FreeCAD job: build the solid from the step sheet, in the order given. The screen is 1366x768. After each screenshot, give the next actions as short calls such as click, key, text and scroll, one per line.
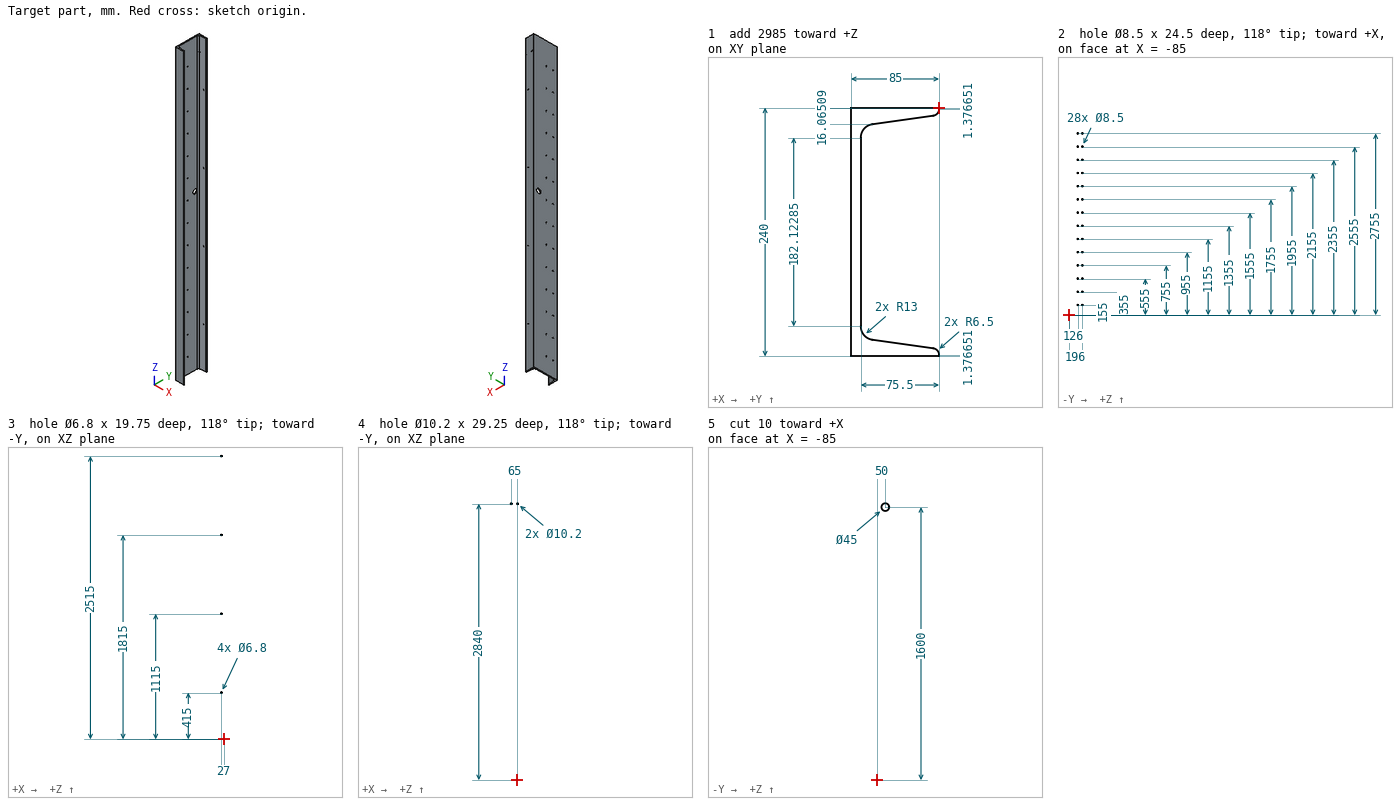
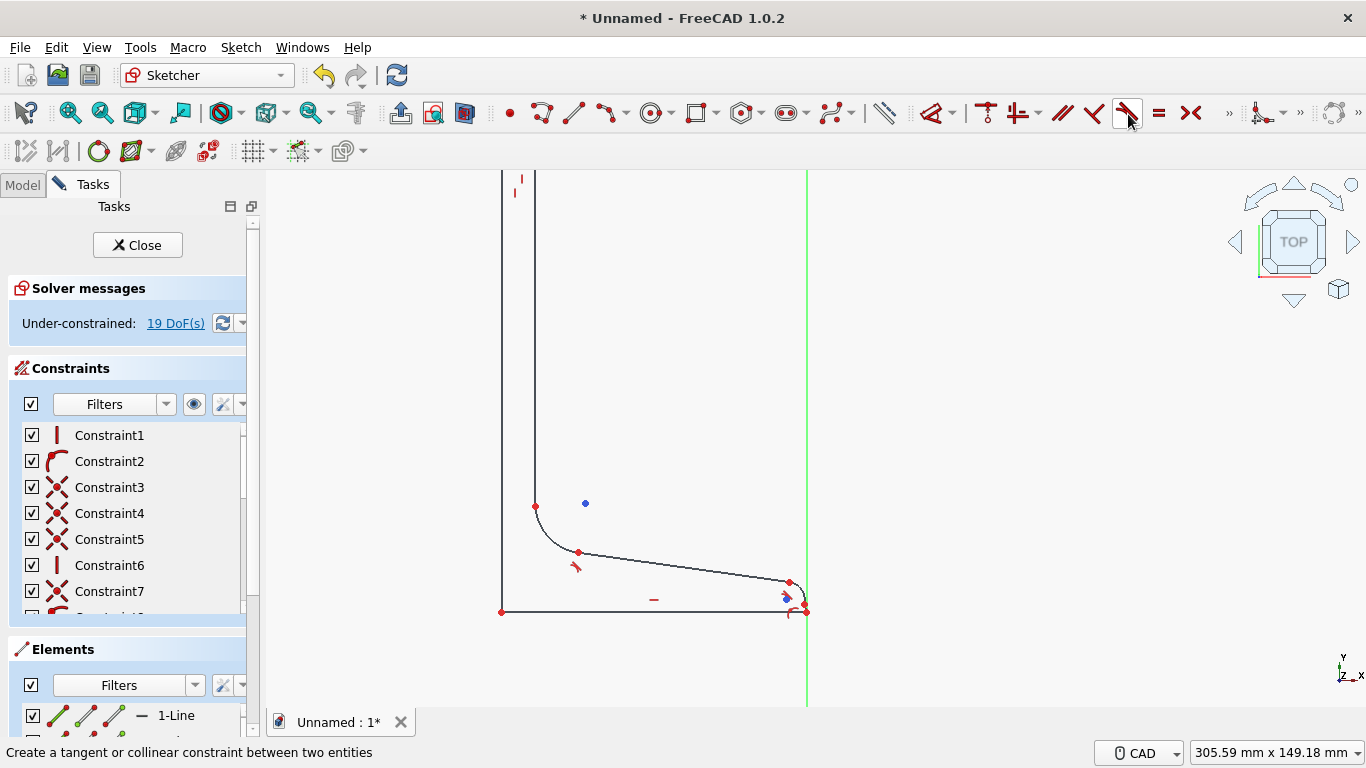
click(535, 310)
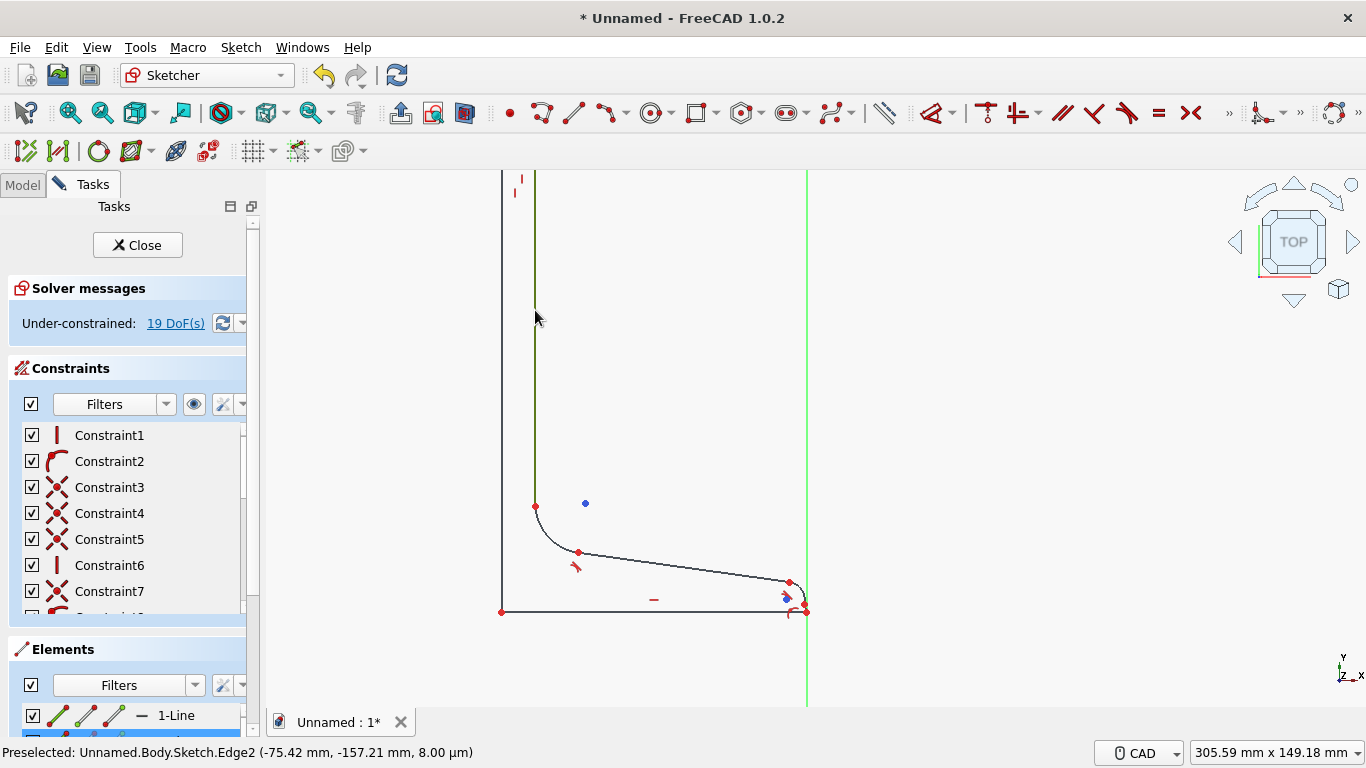
click(541, 526)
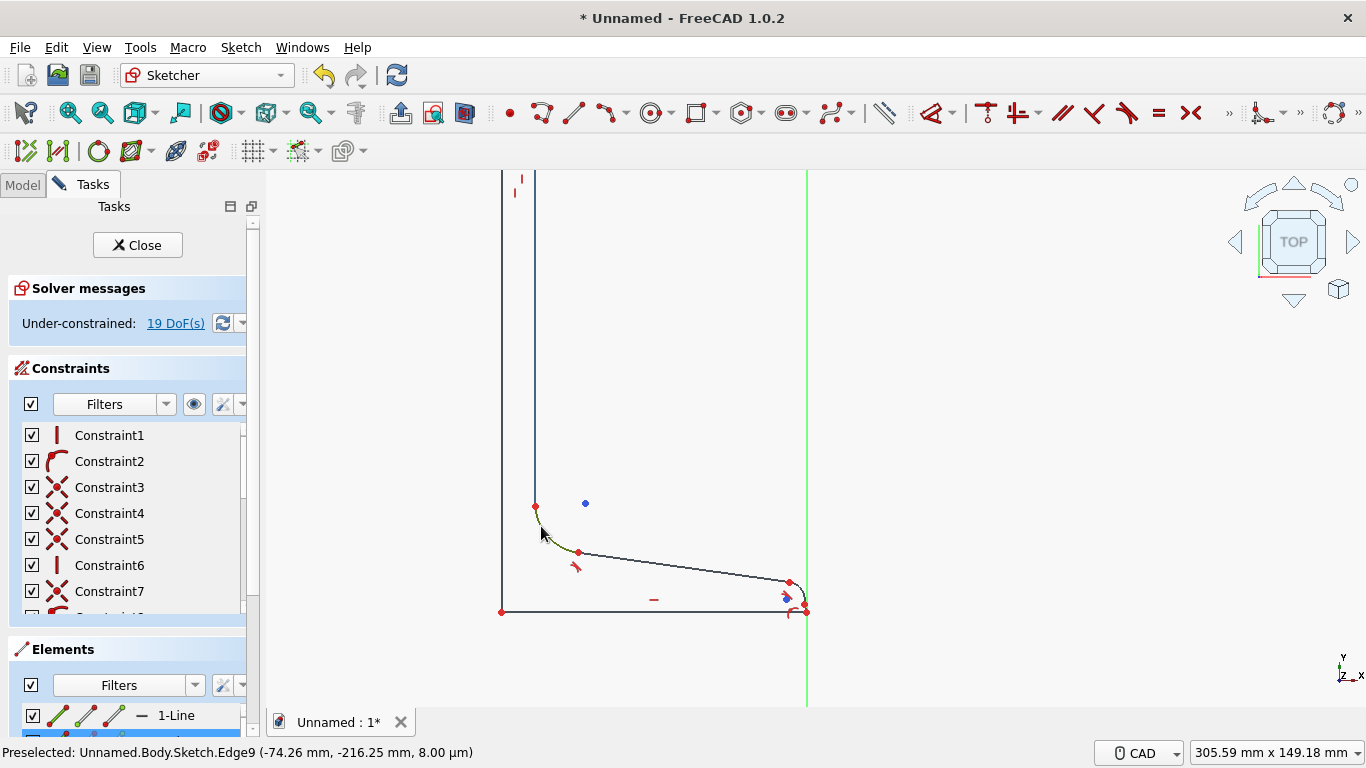
click(1128, 114)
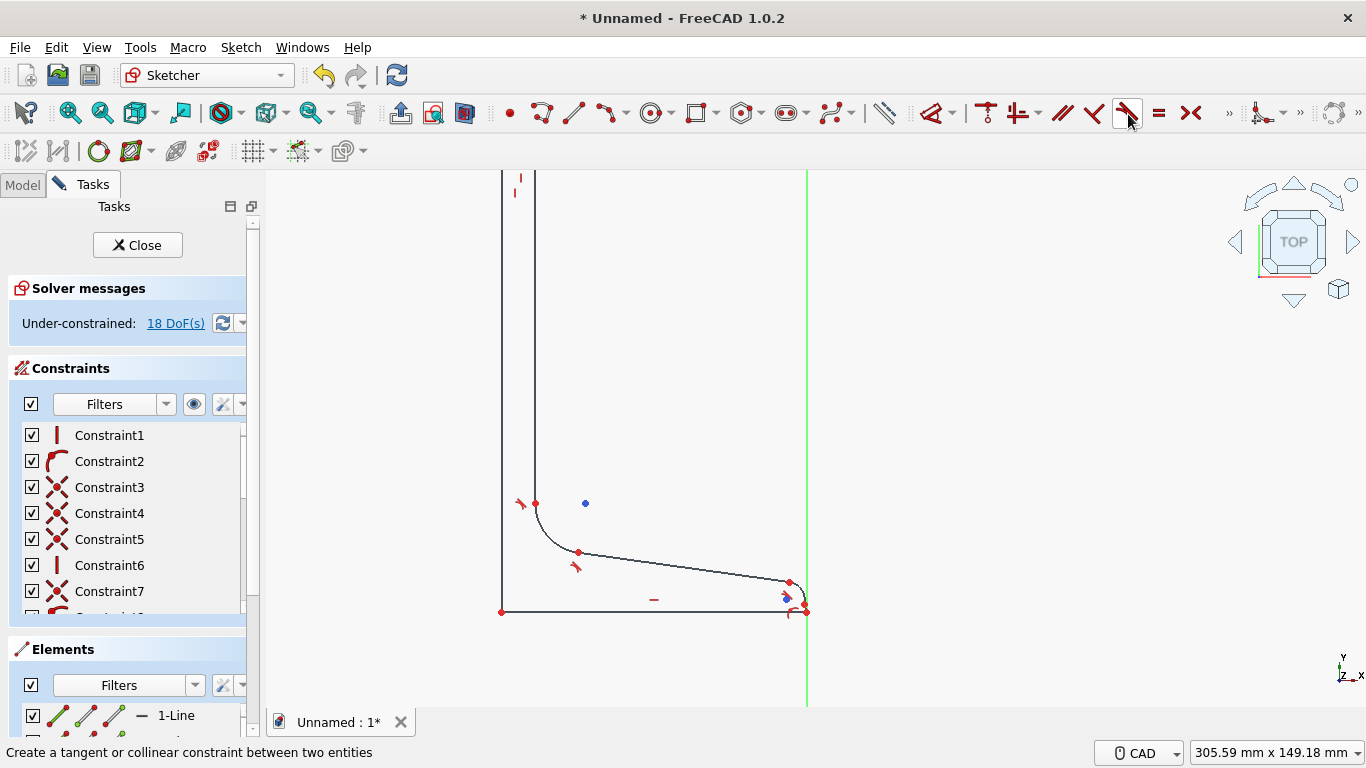
click(535, 308)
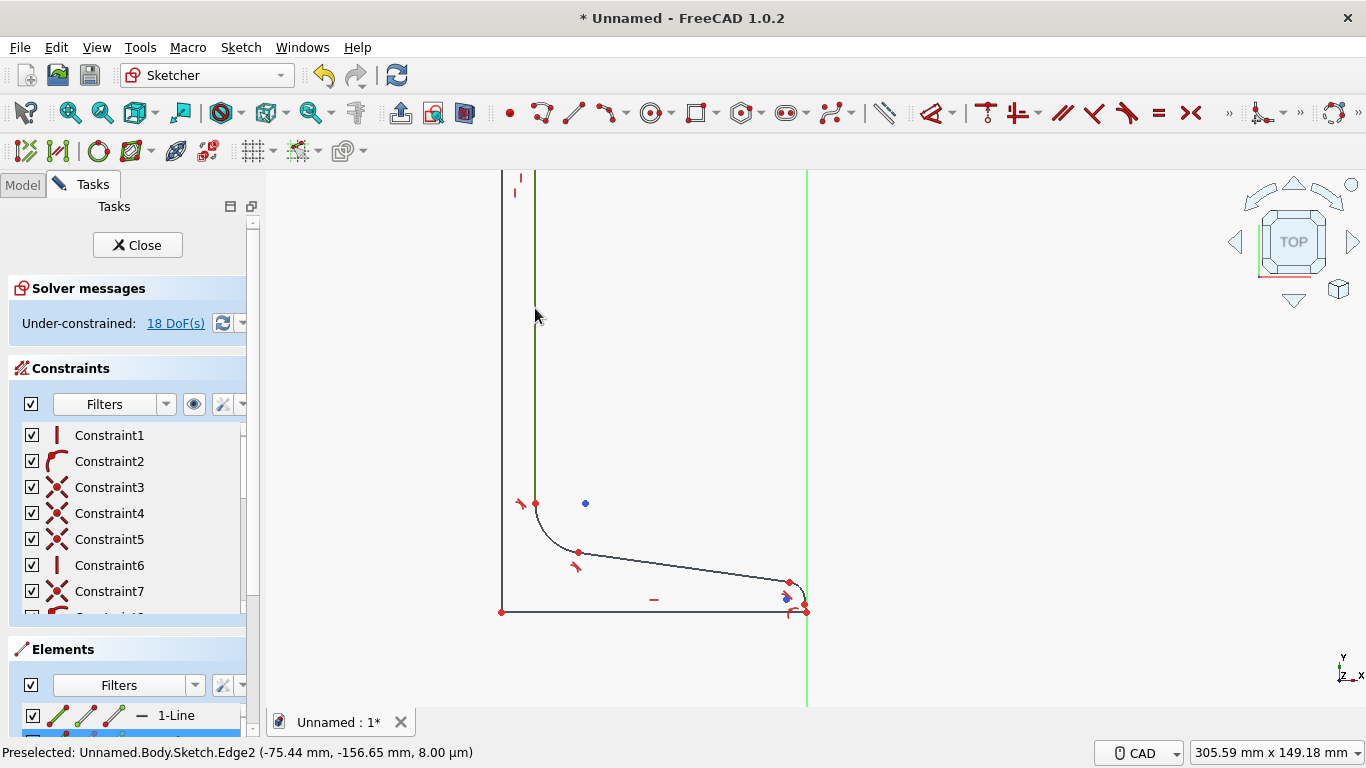
scroll(802, 591, down, 5)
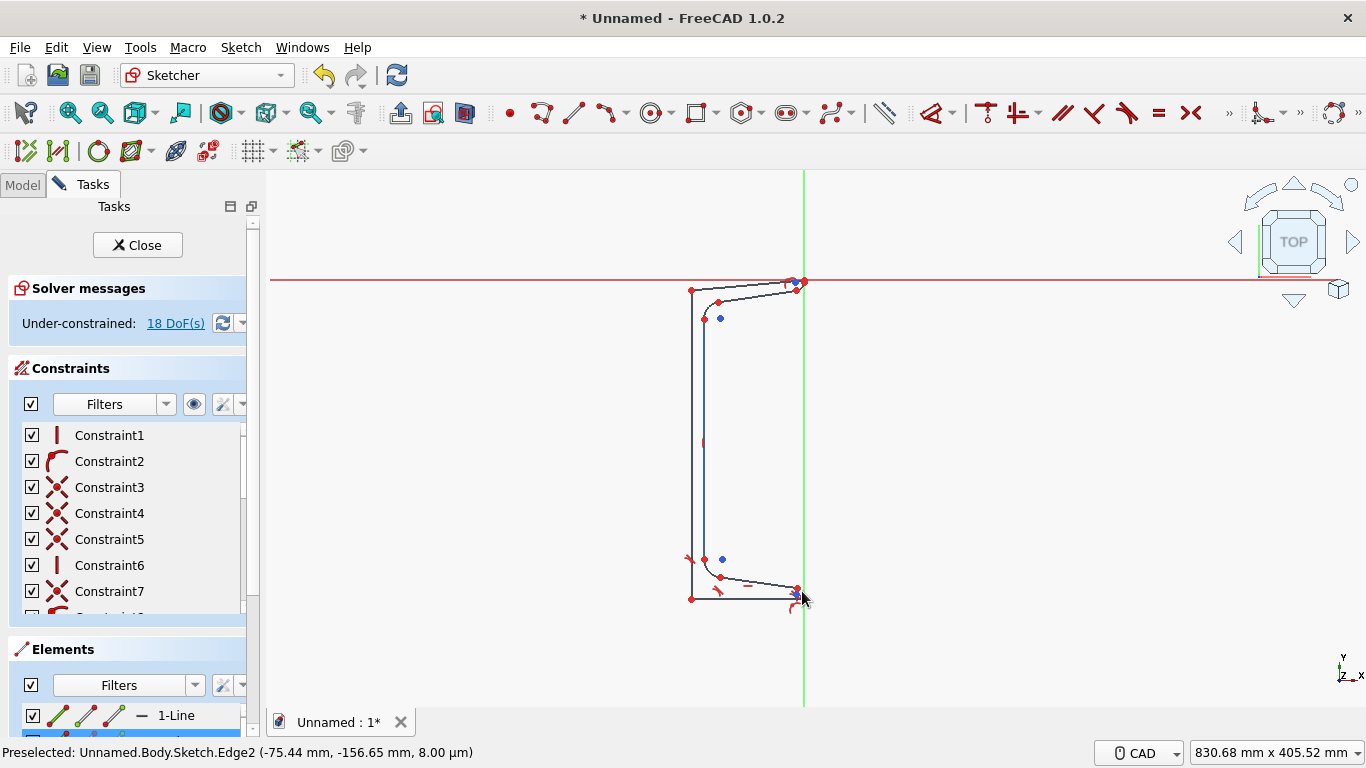
scroll(712, 305, up, 4)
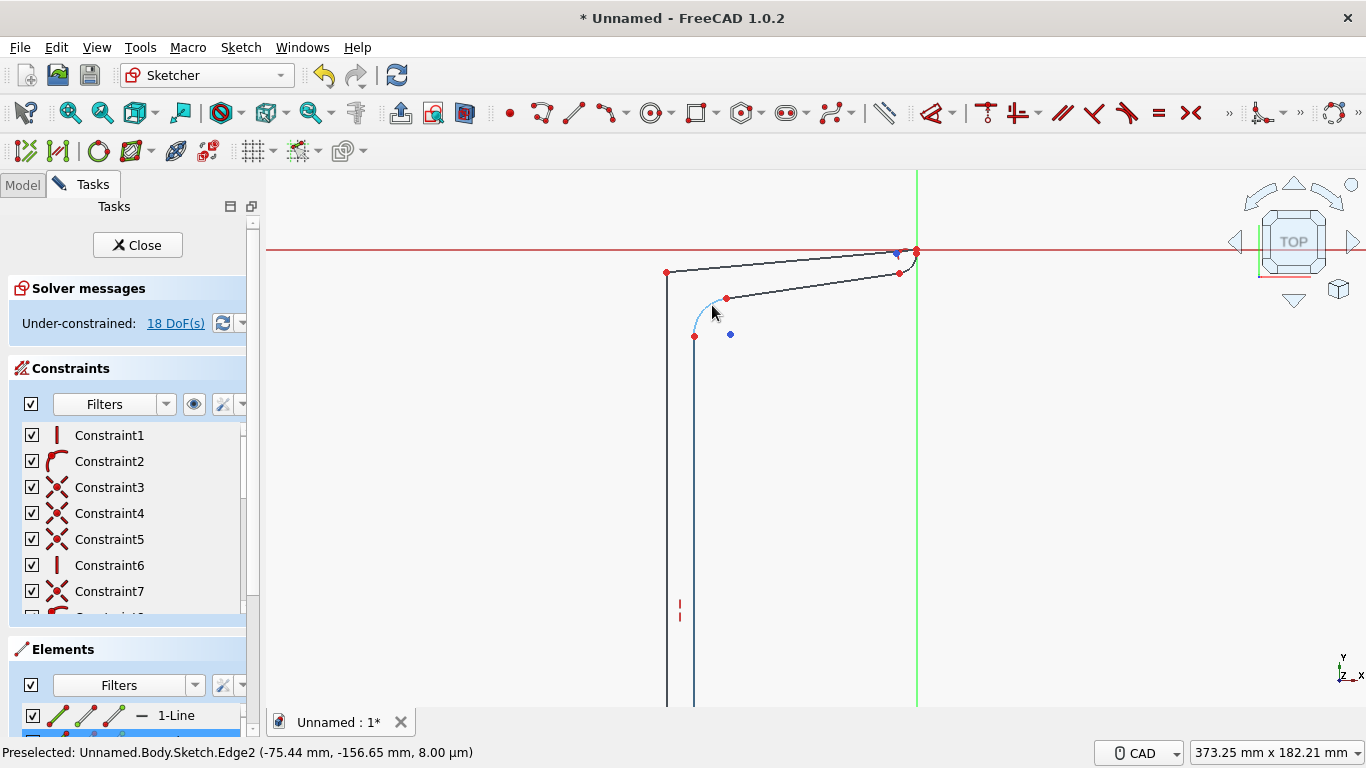
click(711, 304)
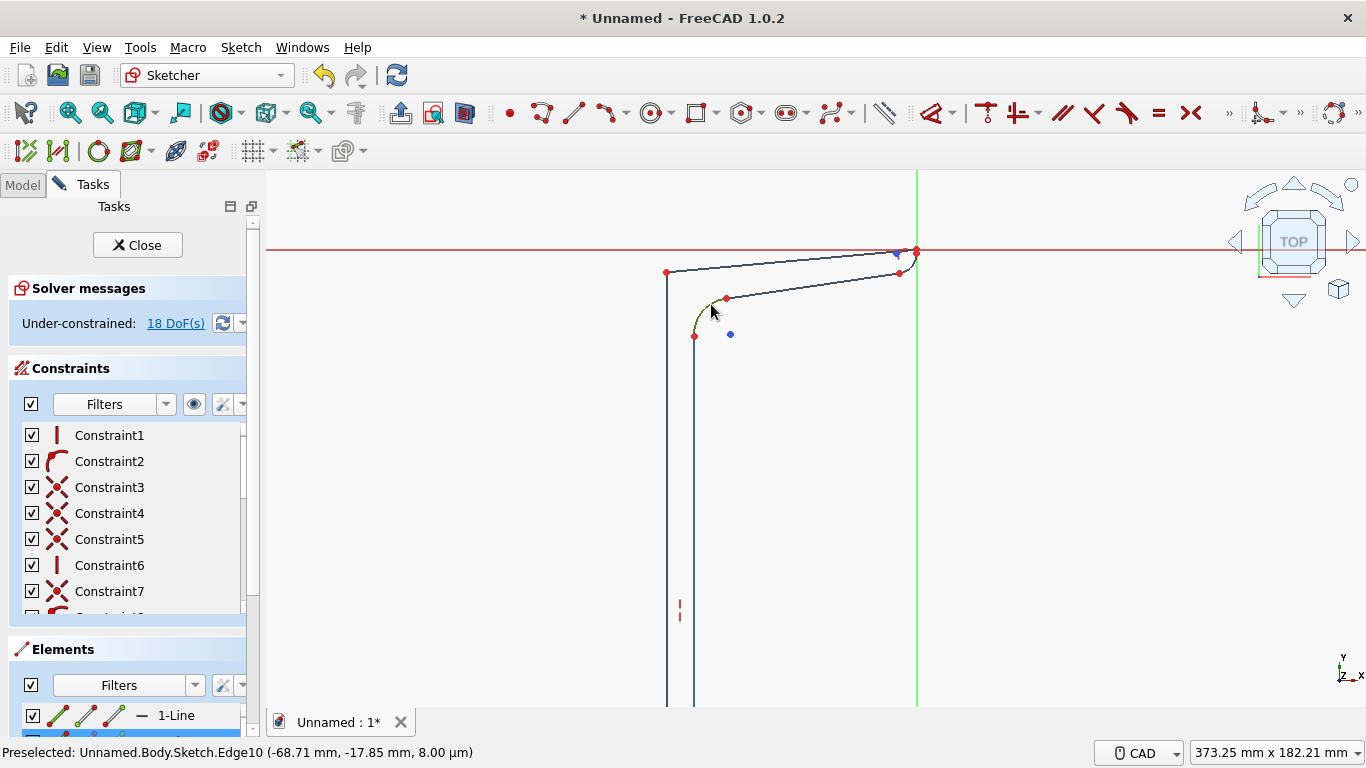
click(1128, 114)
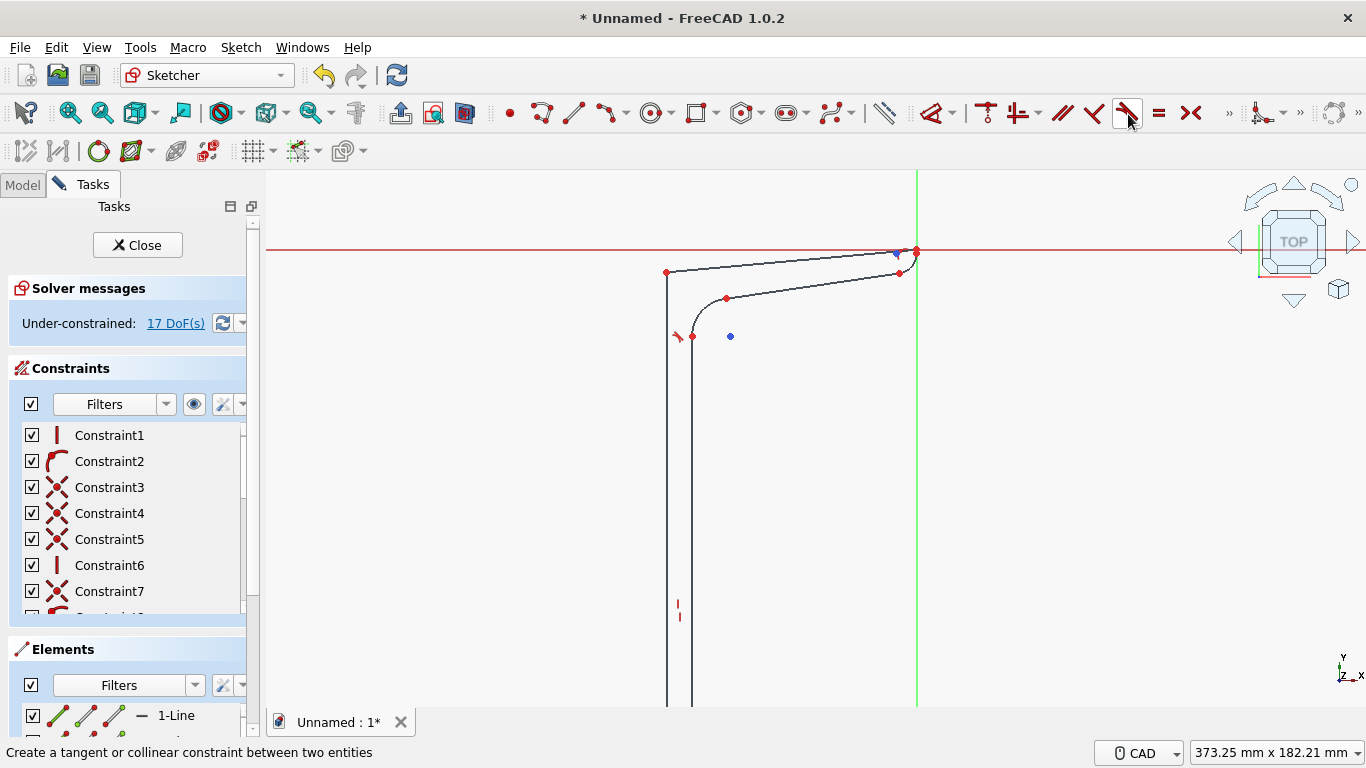
click(779, 291)